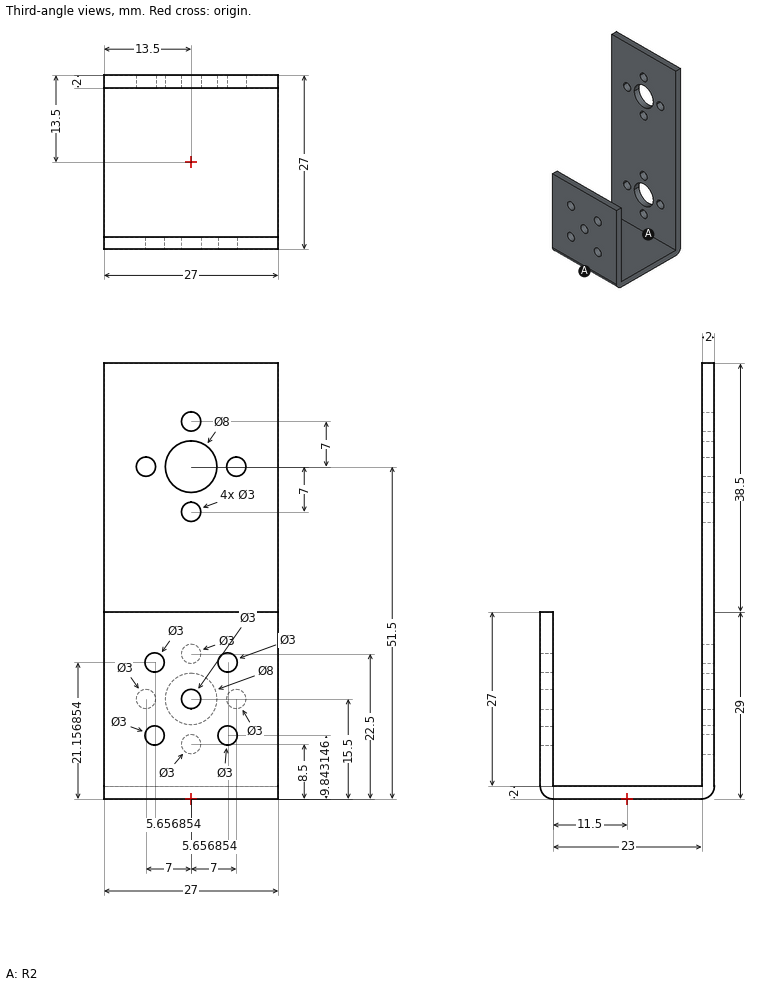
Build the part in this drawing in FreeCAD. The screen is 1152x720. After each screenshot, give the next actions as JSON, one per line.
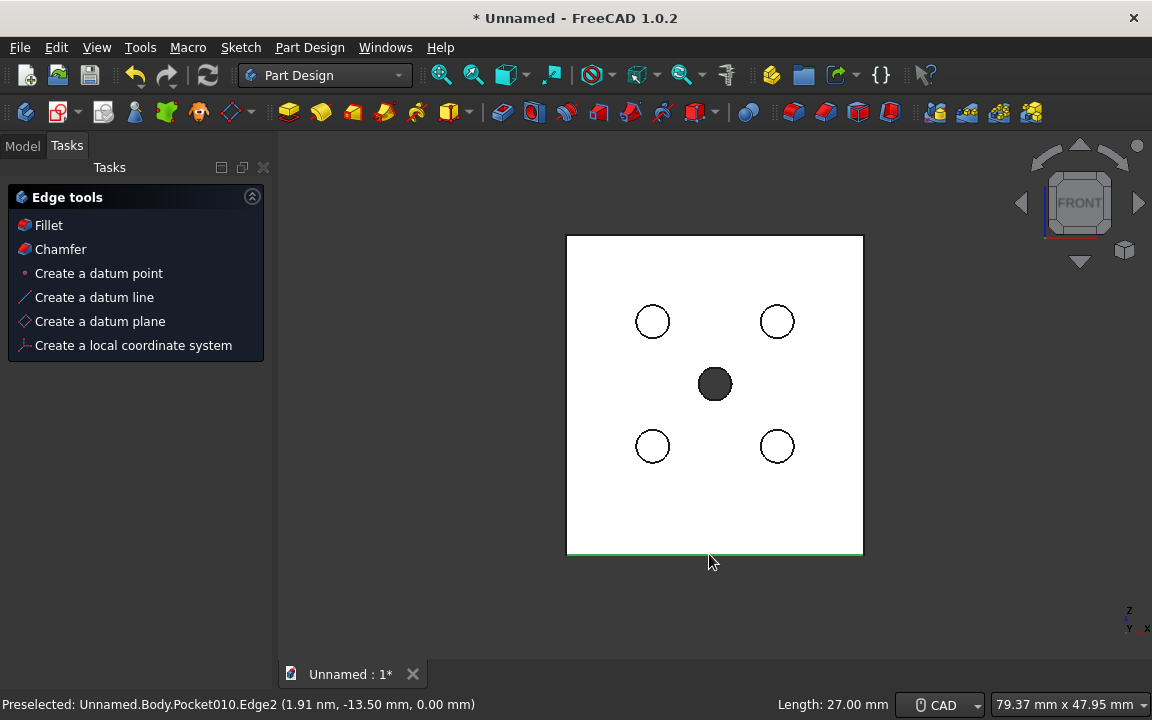
{"action": "key", "text": "3"}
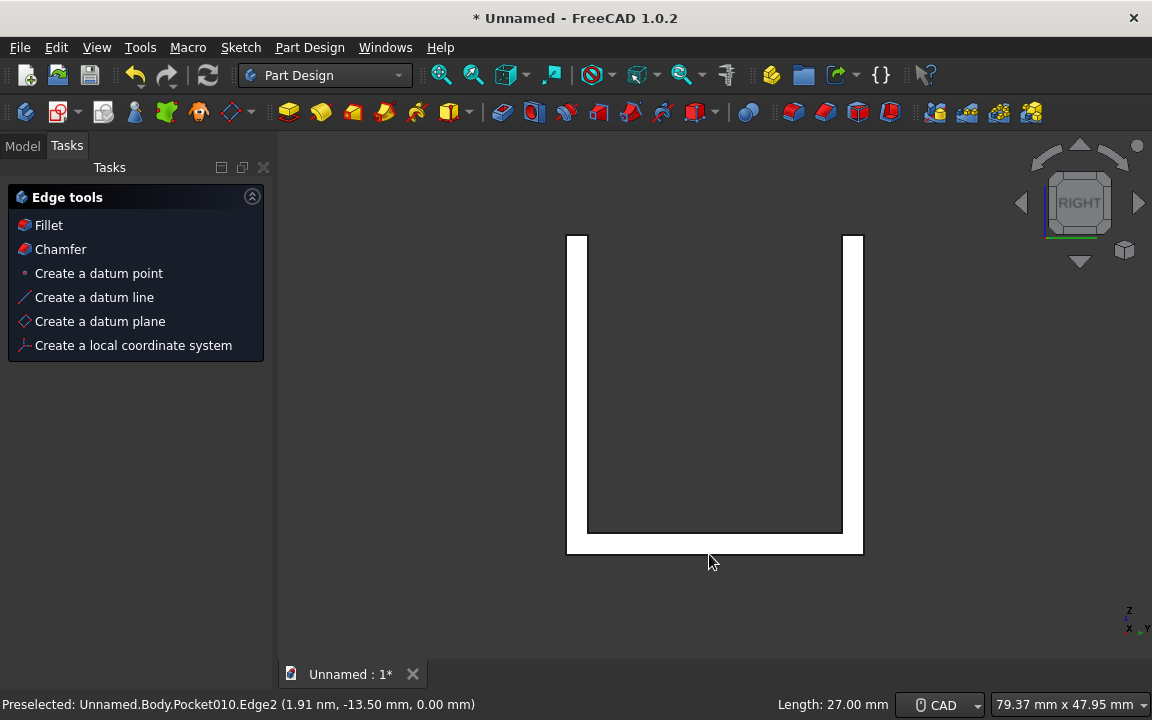
{"action": "key", "text": "5"}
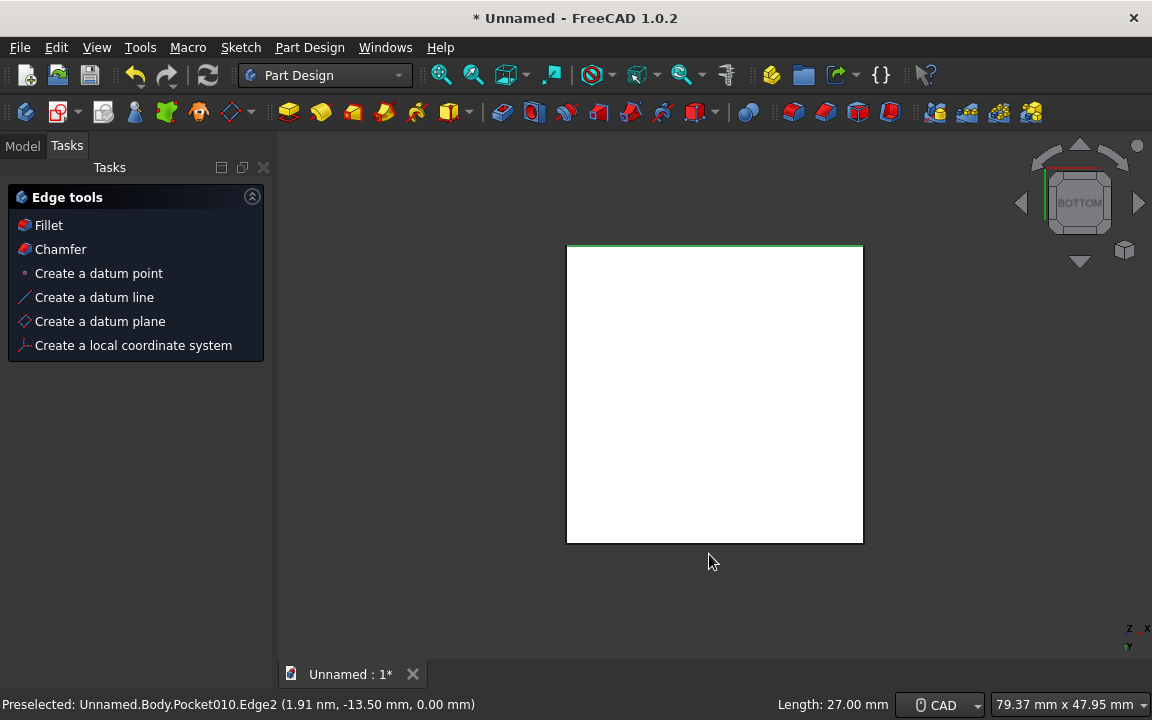
{"action": "left_click", "coordinate": [715, 543], "text": "ctrl"}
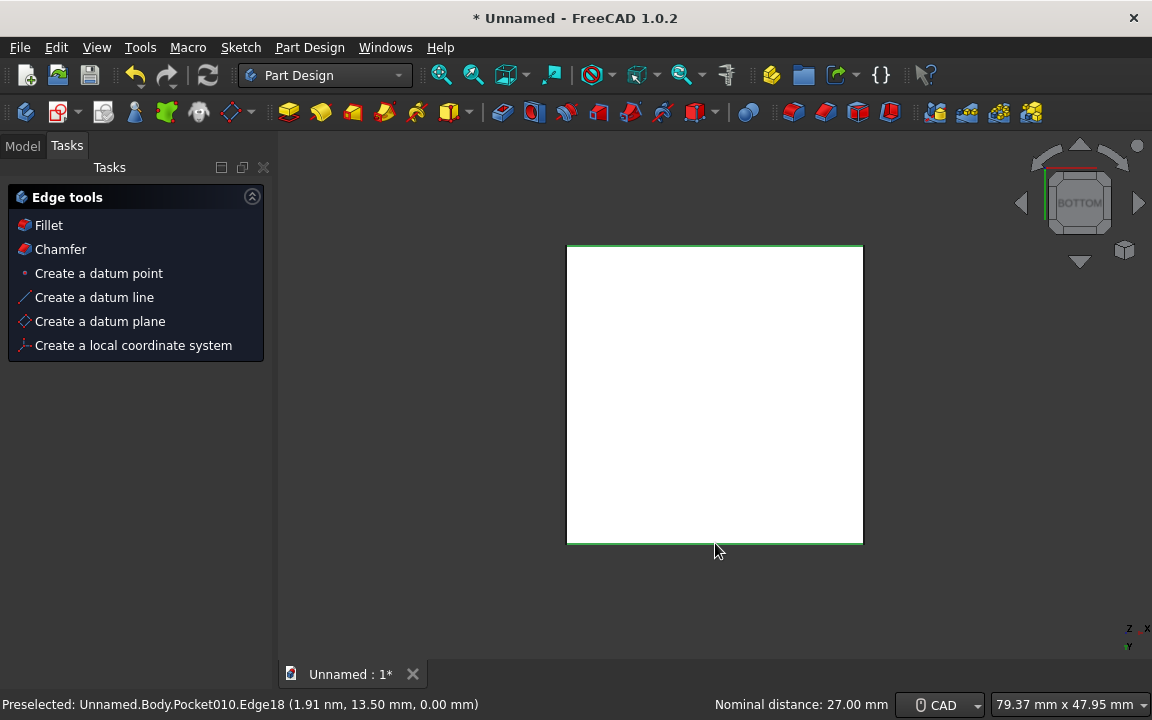
{"action": "left_click", "coordinate": [794, 112]}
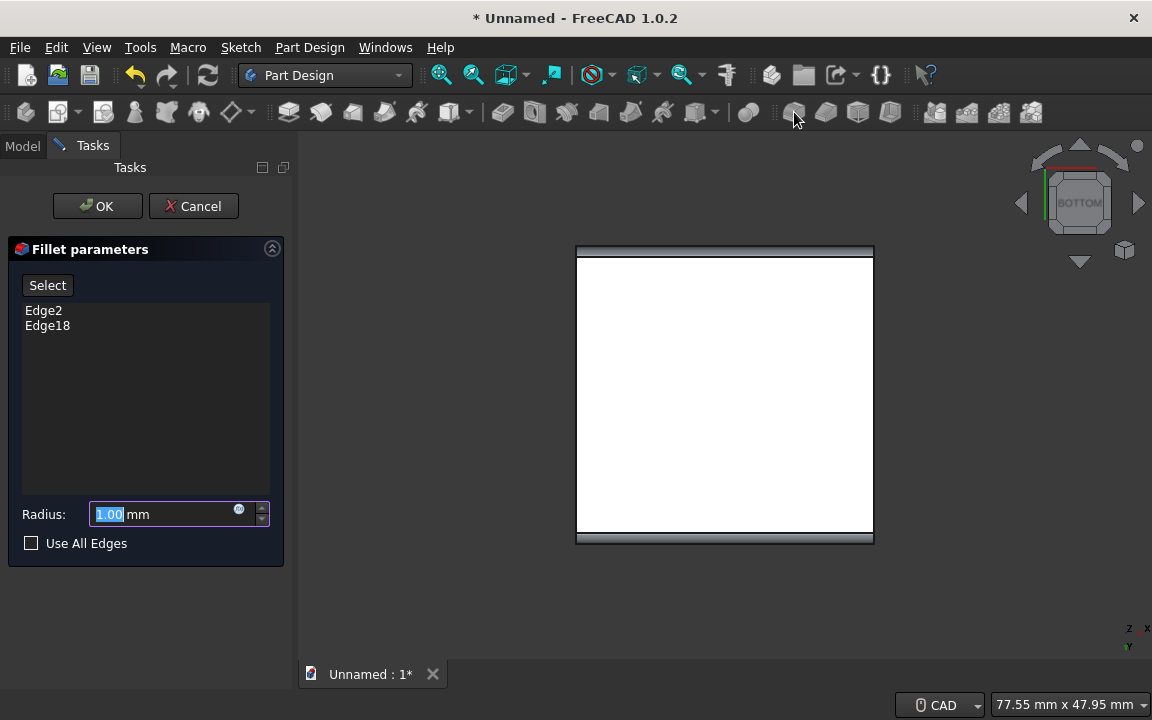
{"action": "type", "text": "2"}
{"action": "key", "text": "Tab"}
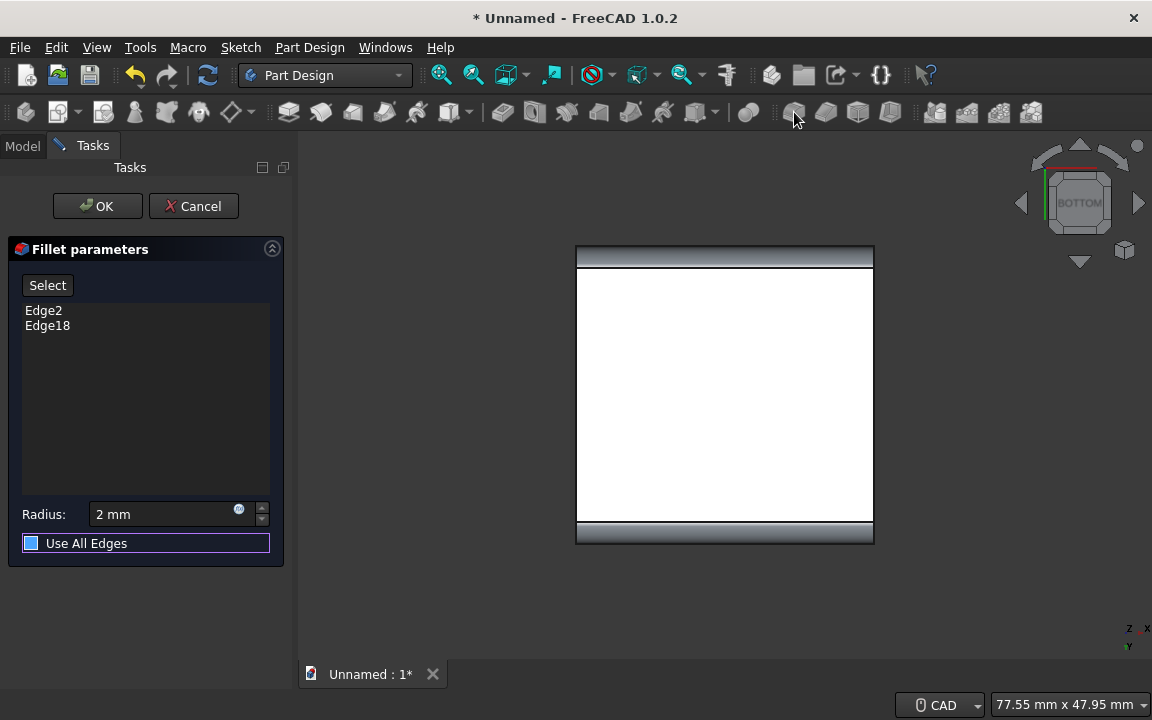
{"action": "left_click", "coordinate": [98, 206]}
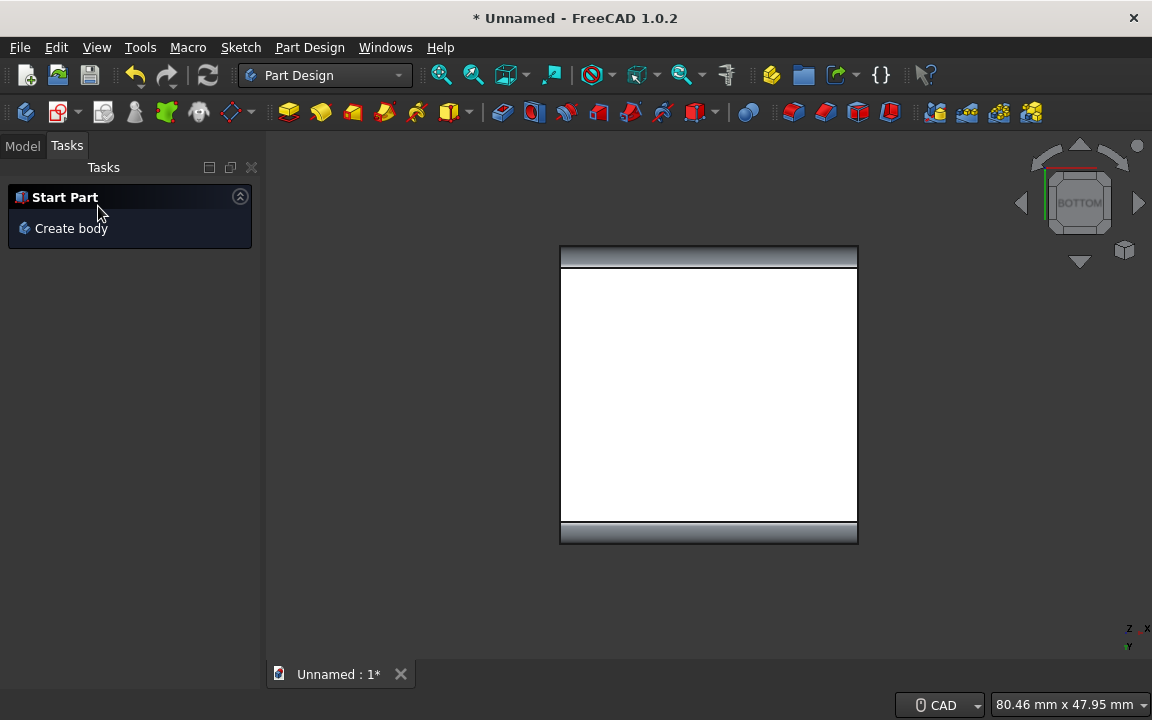
{"action": "key", "text": "0"}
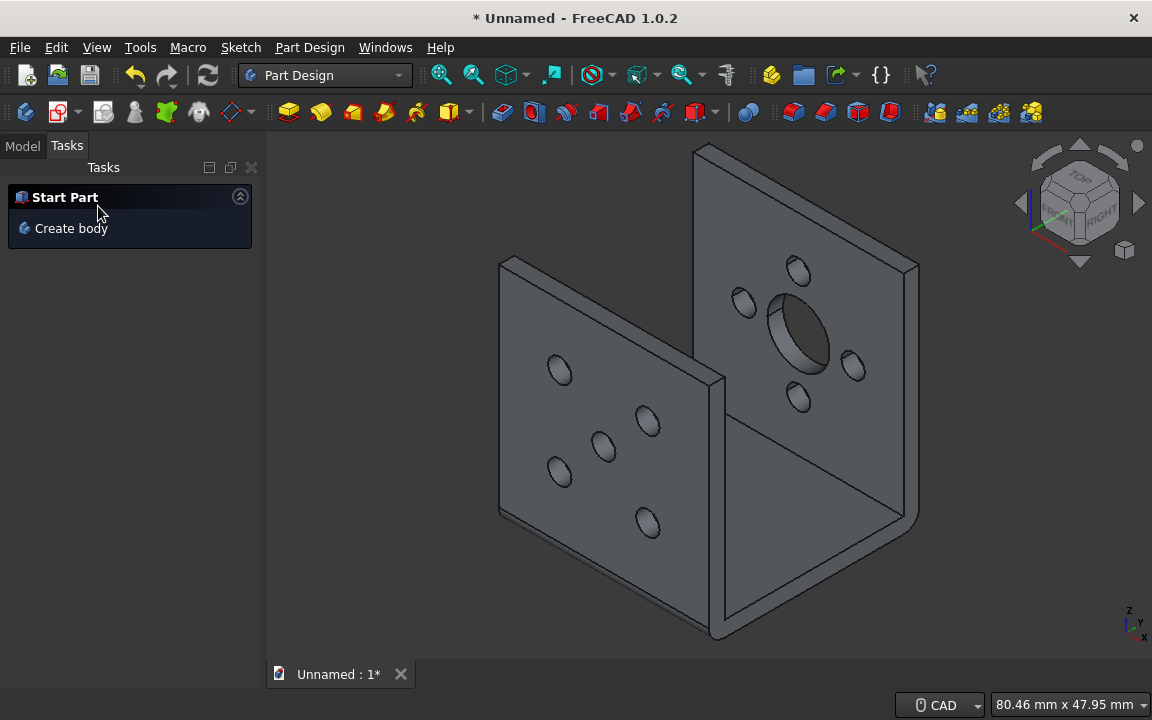
{"action": "left_click", "coordinate": [704, 371]}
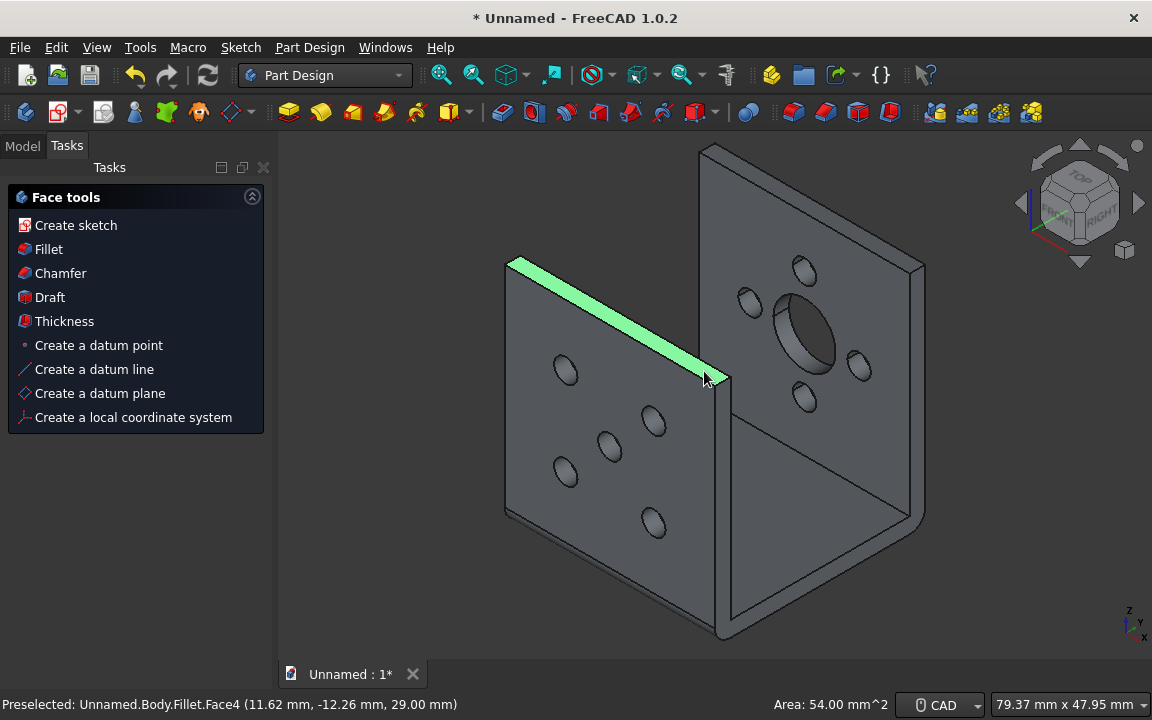
{"action": "left_click", "coordinate": [58, 112]}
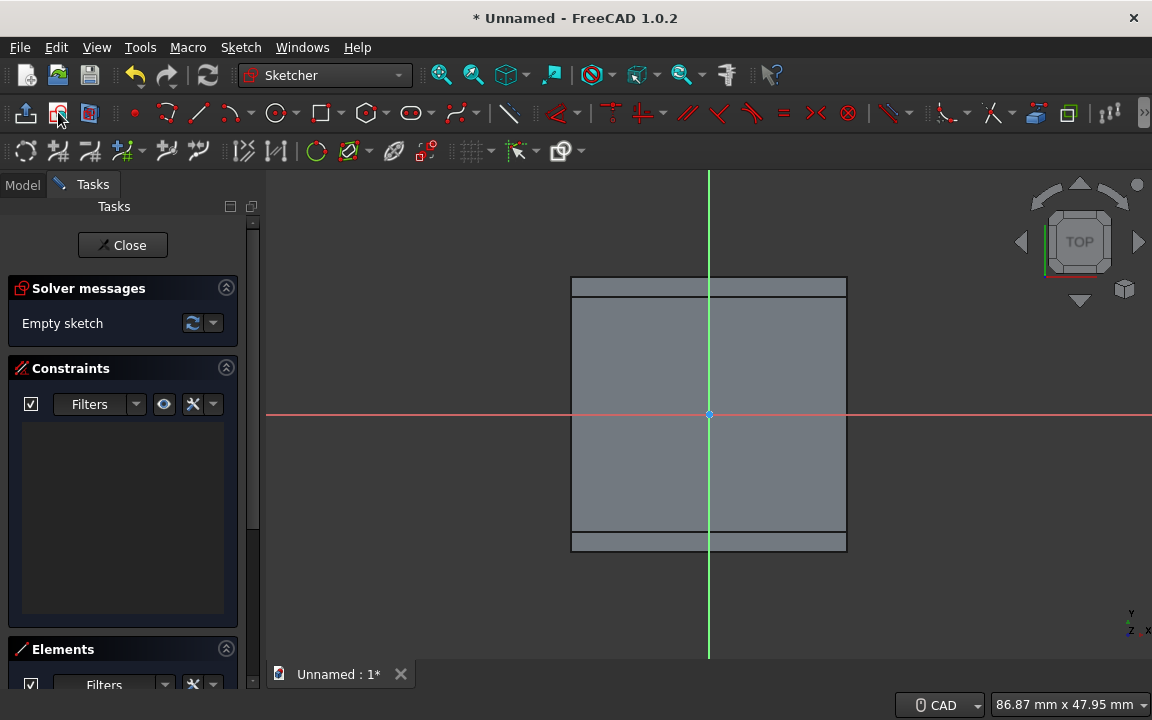
{"action": "scroll", "coordinate": [792, 262], "scroll_direction": "up", "scroll_amount": 3}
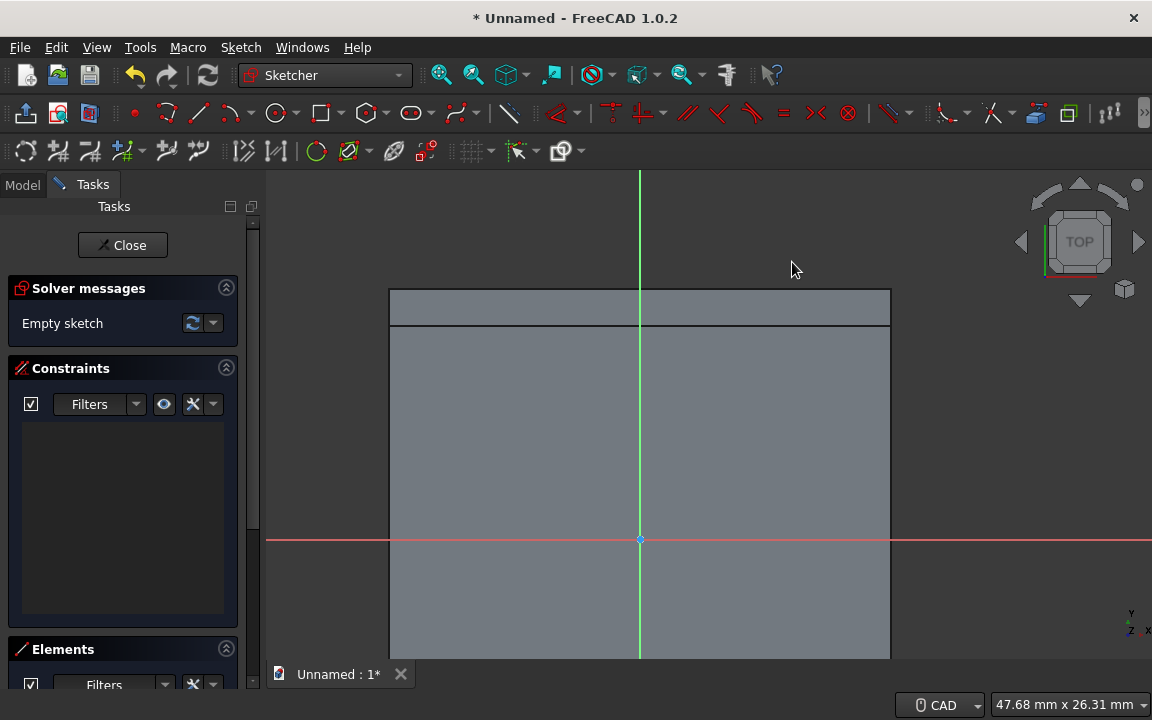
{"action": "key", "text": "g r"}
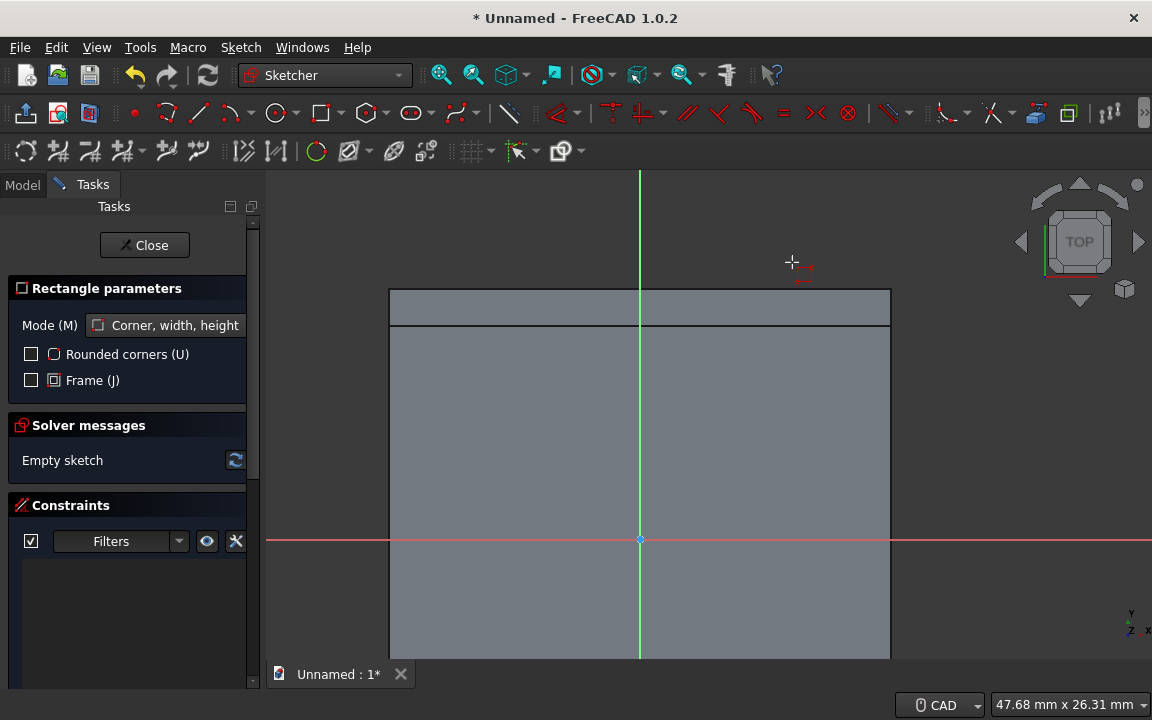
{"action": "left_click", "coordinate": [389, 289]}
{"action": "left_click", "coordinate": [891, 326]}
{"action": "key", "text": "Escape"}